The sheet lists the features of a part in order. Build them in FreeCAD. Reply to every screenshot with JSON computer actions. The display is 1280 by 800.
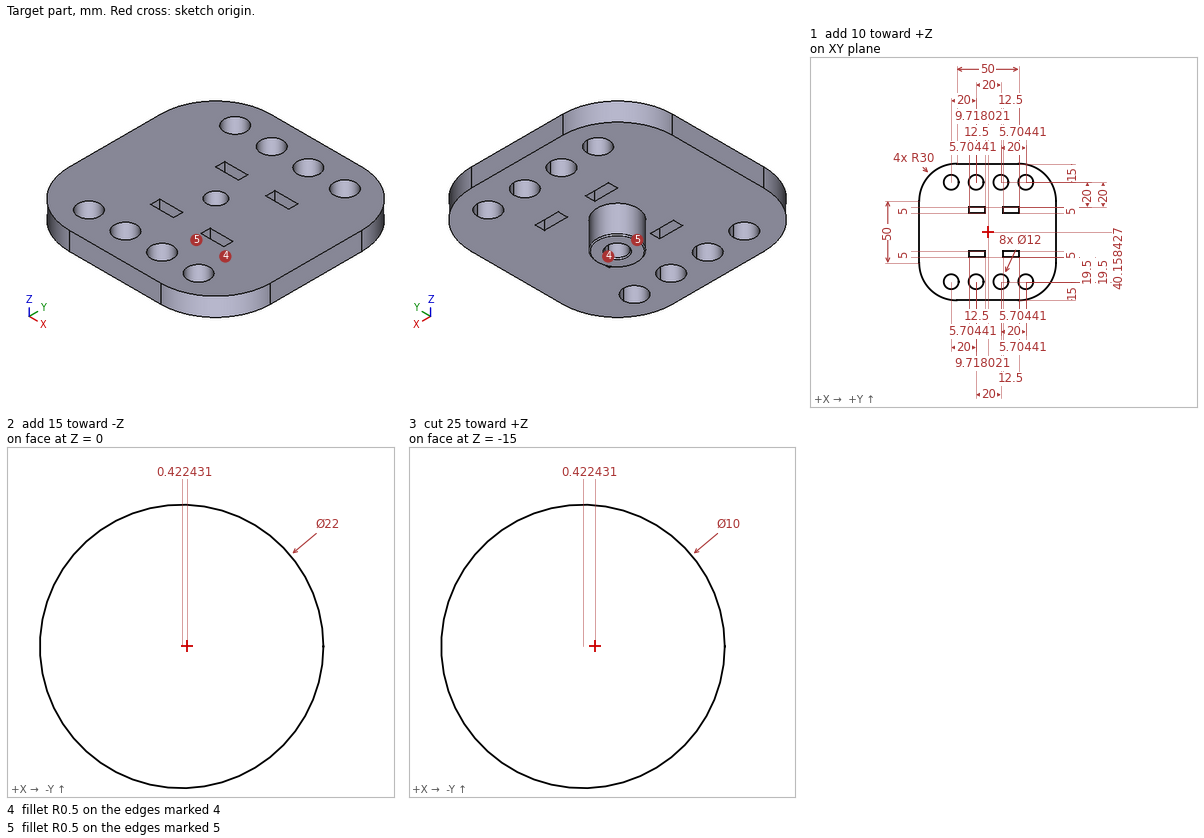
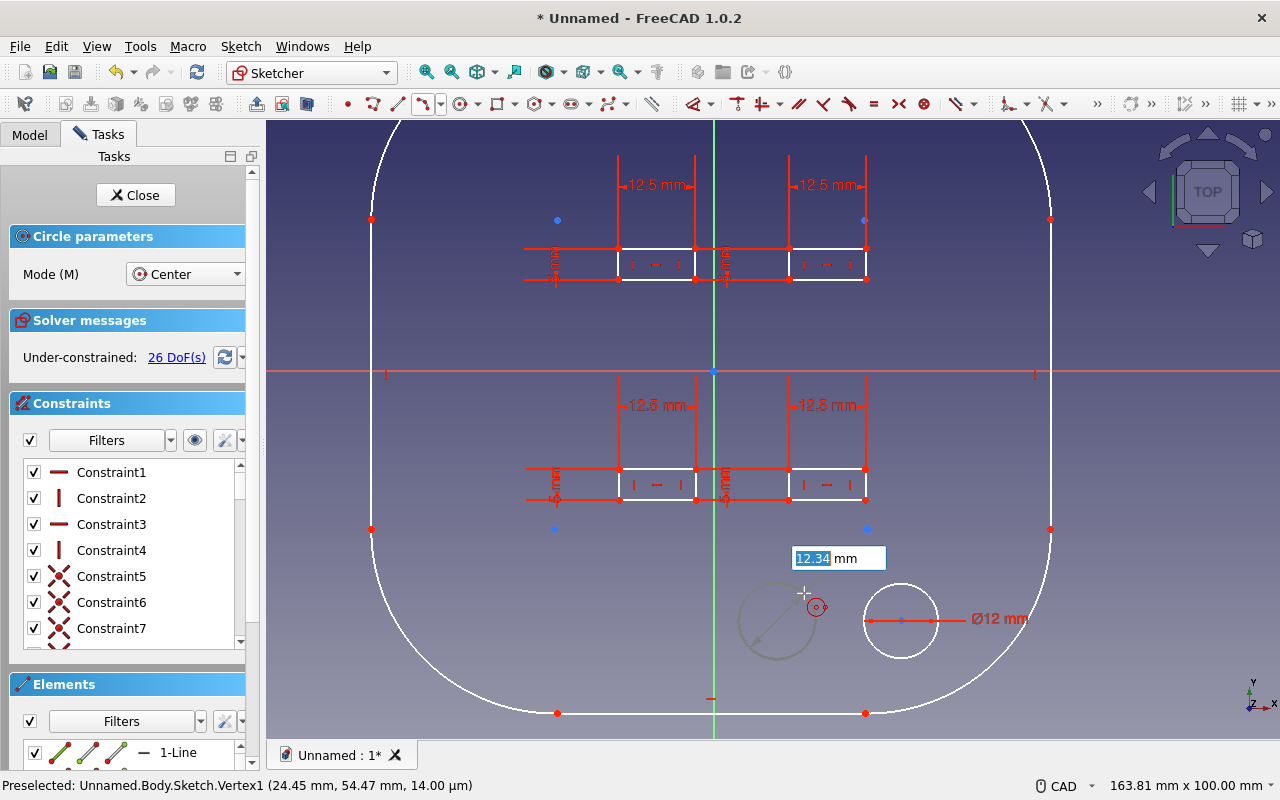
{"action": "type", "text": "12"}
{"action": "key", "text": "Return"}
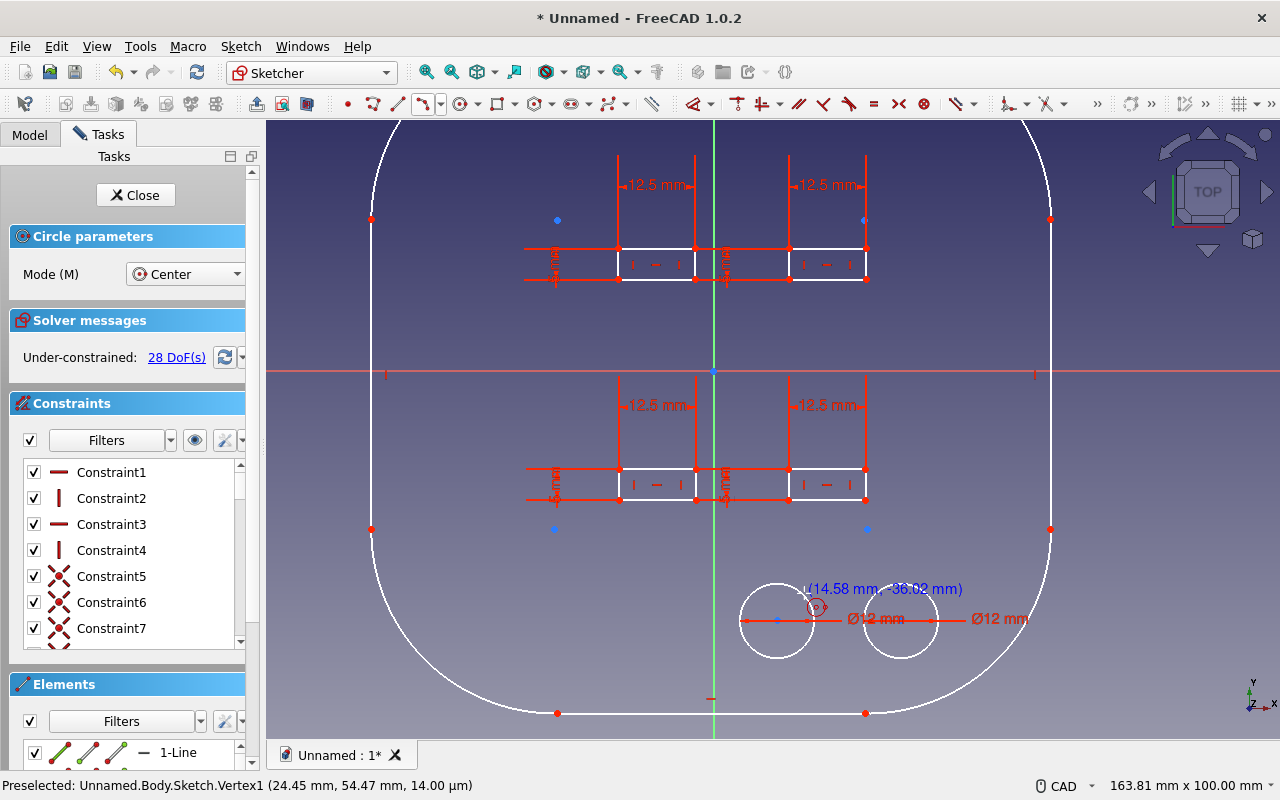
{"action": "left_click", "coordinate": [654, 620]}
{"action": "mouse_move", "coordinate": [680, 593]}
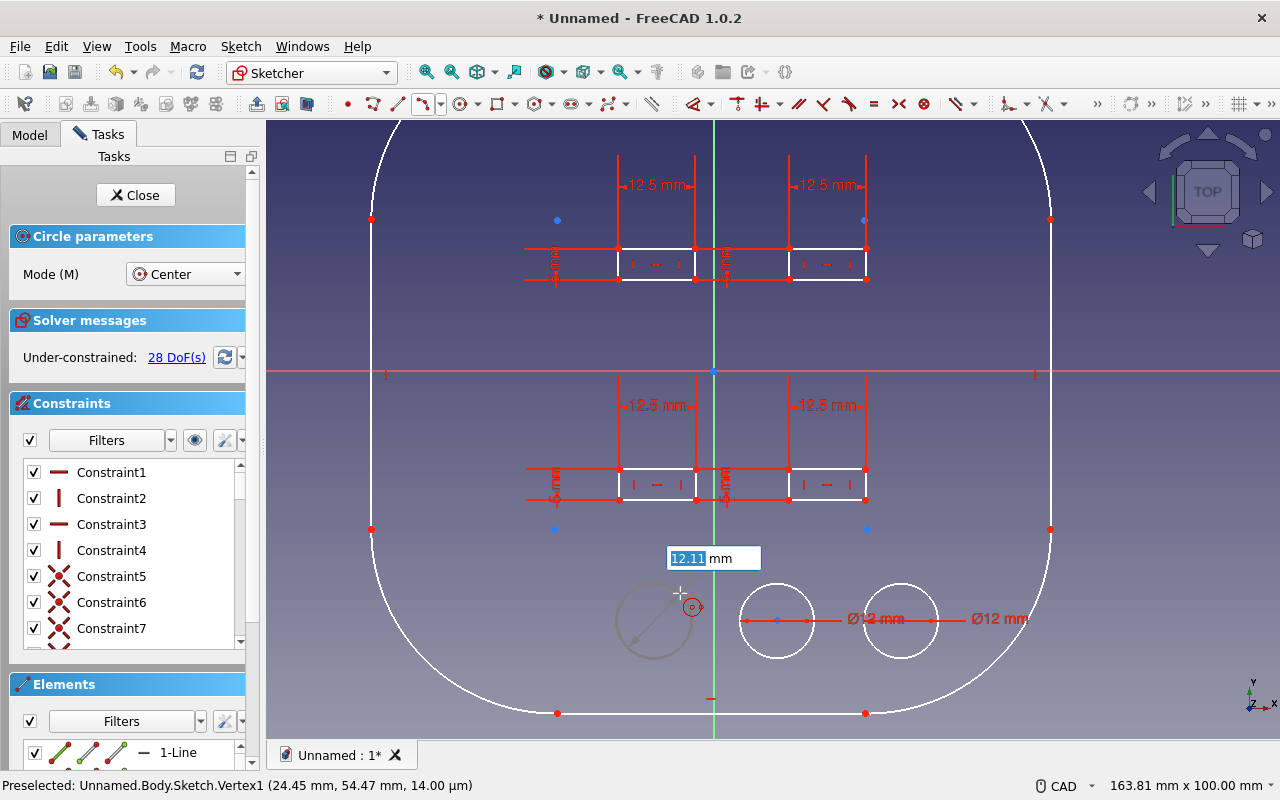
{"action": "type", "text": "12"}
{"action": "key", "text": "Return"}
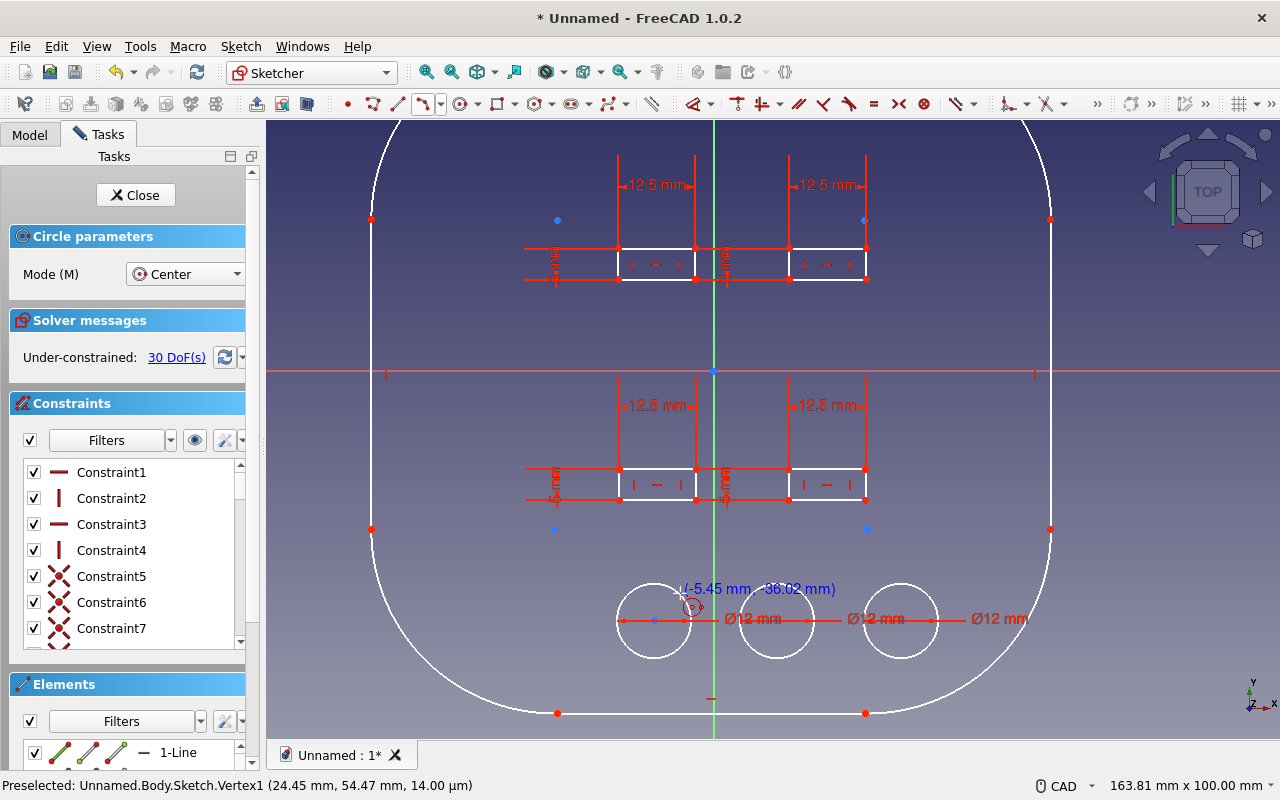
{"action": "left_click", "coordinate": [530, 620]}
{"action": "mouse_move", "coordinate": [556, 593]}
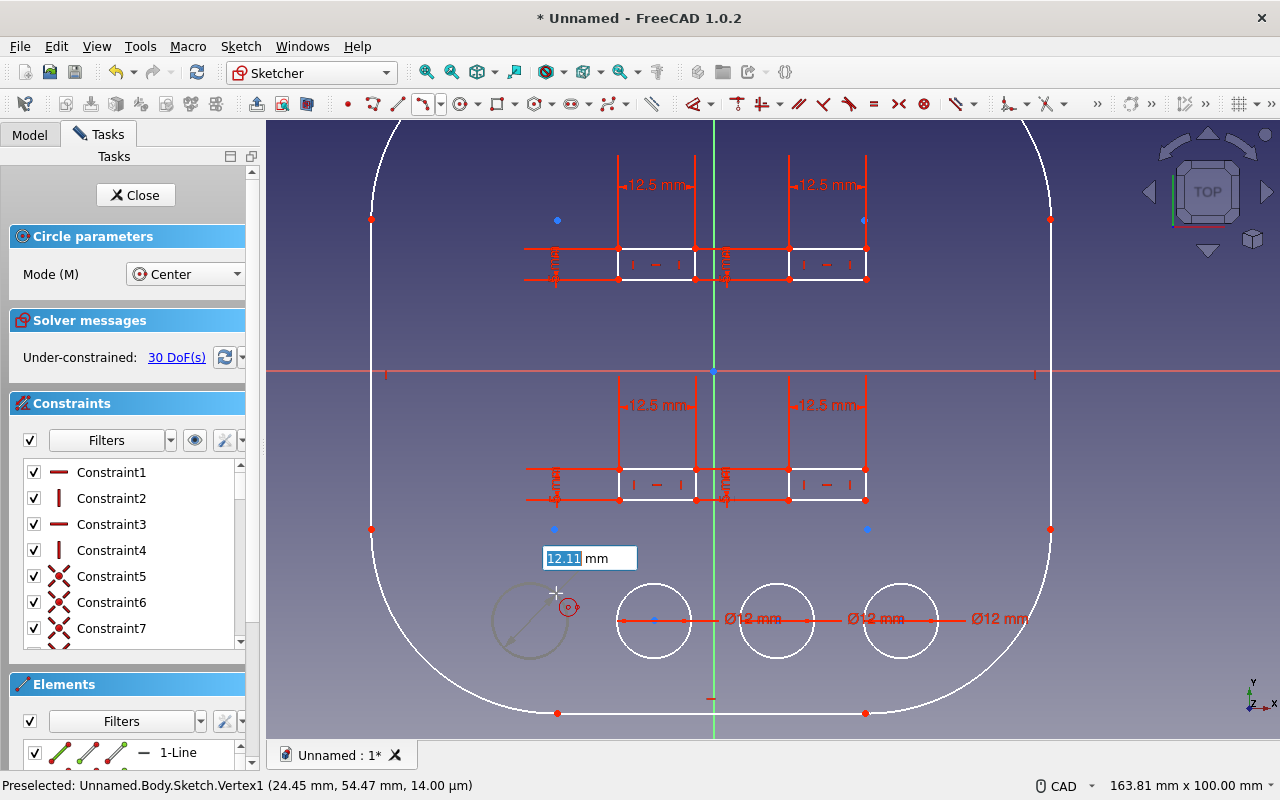
{"action": "type", "text": "12"}
{"action": "key", "text": "Return"}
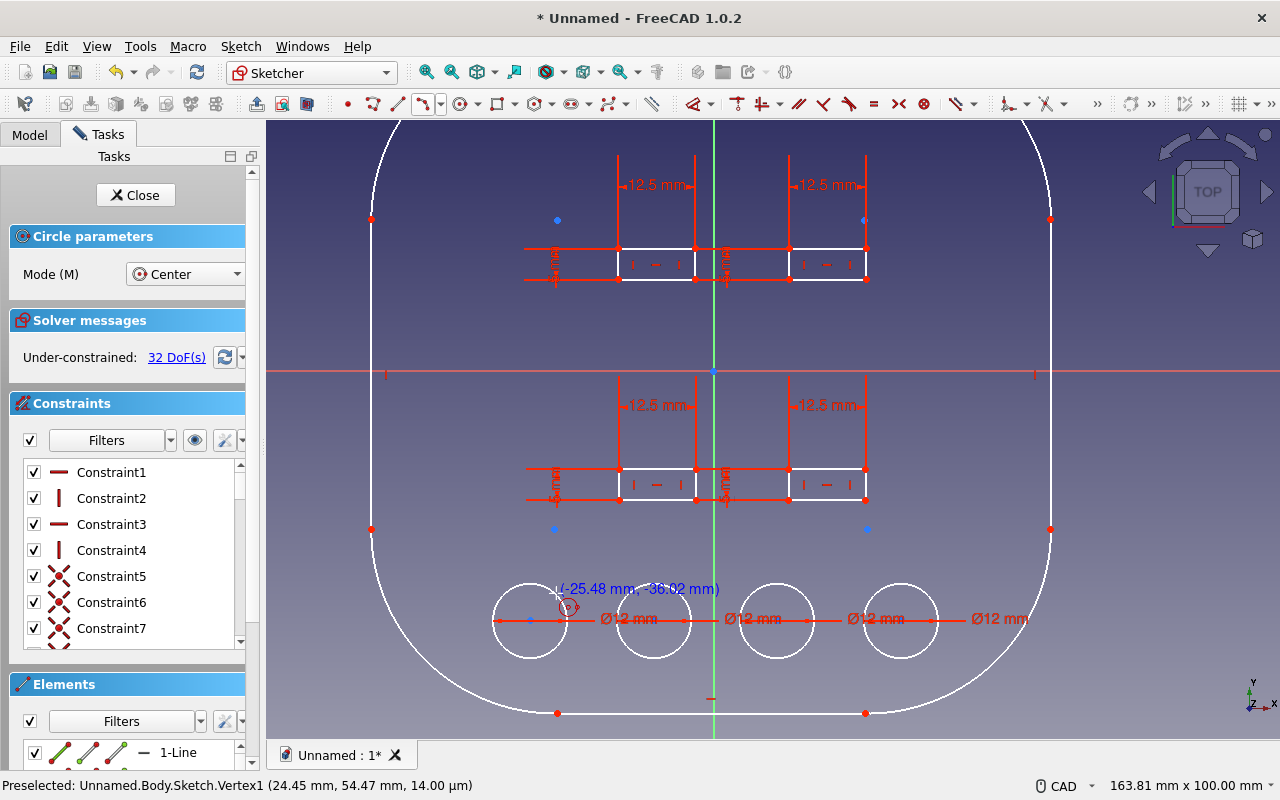
{"action": "scroll", "coordinate": [696, 499], "scroll_direction": "down", "scroll_amount": 3}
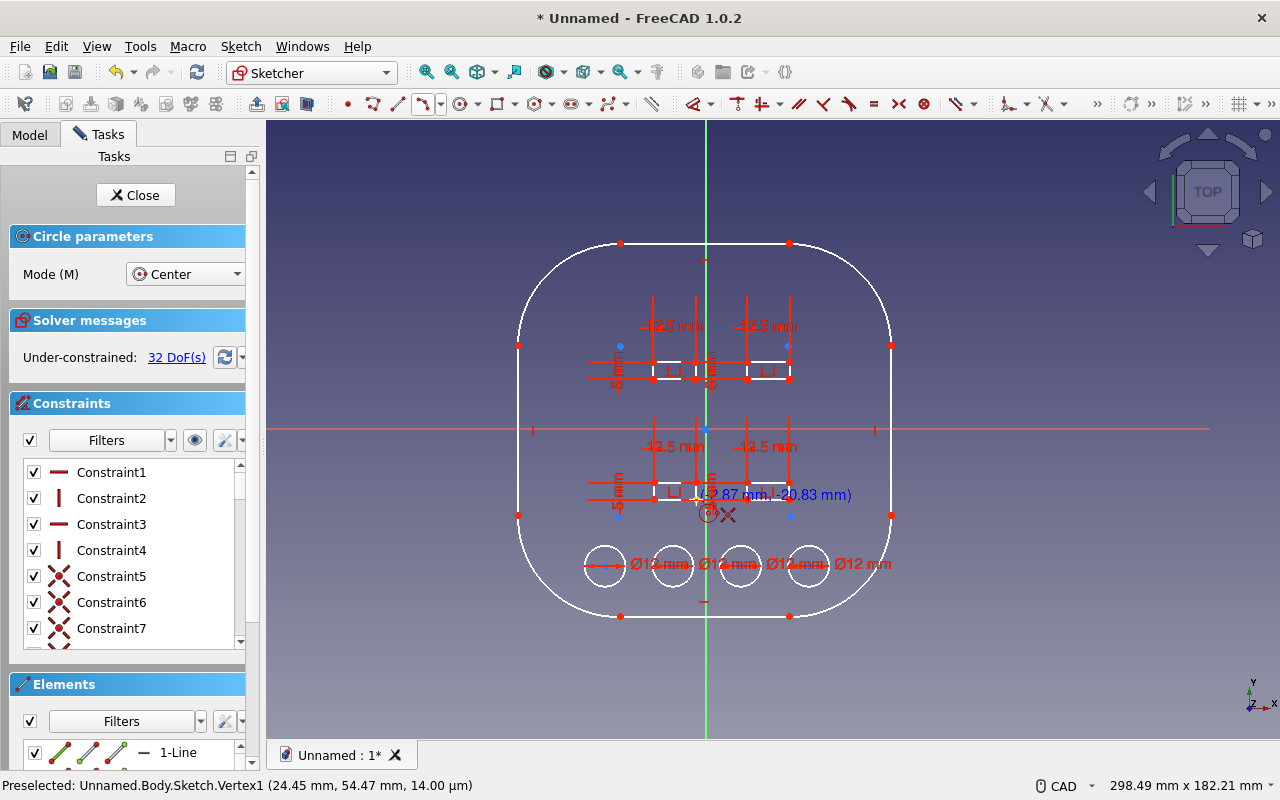
{"action": "left_click", "coordinate": [809, 294]}
{"action": "mouse_move", "coordinate": [823, 279]}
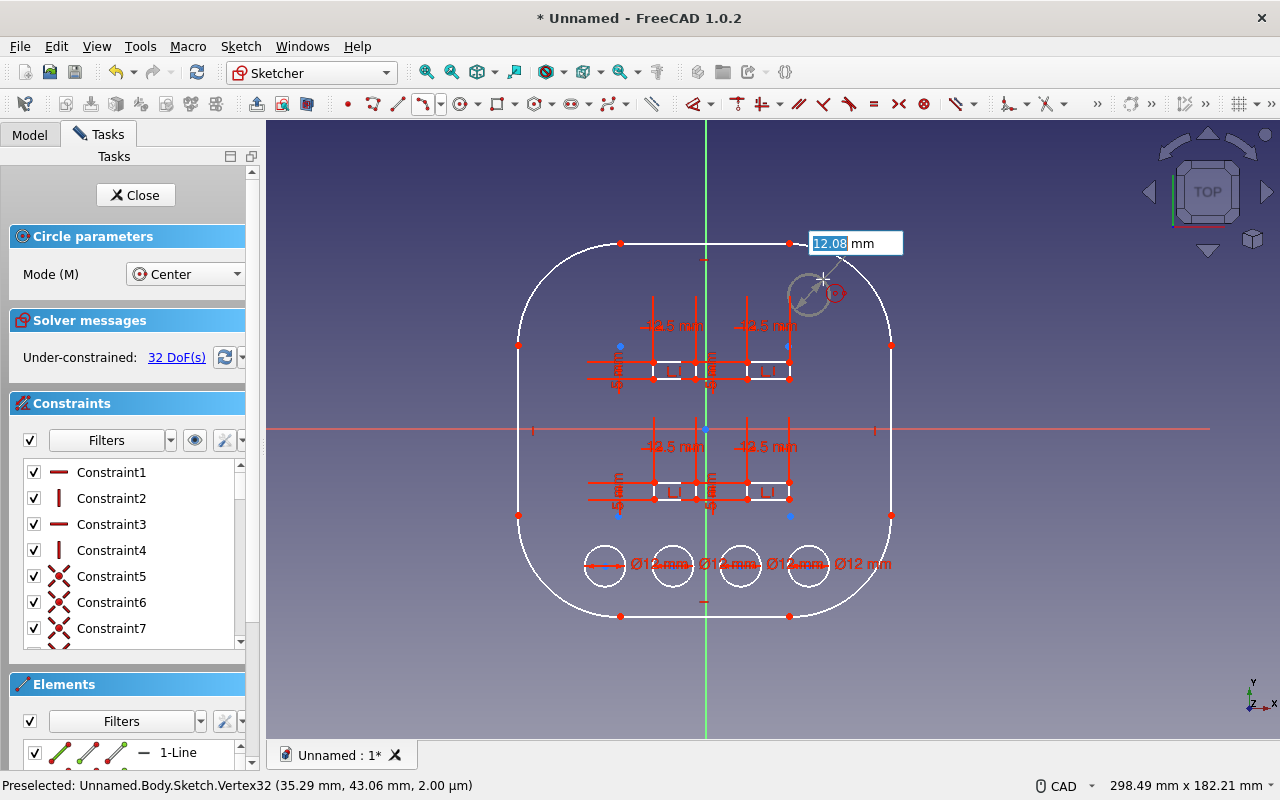
{"action": "type", "text": "12"}
{"action": "key", "text": "Return"}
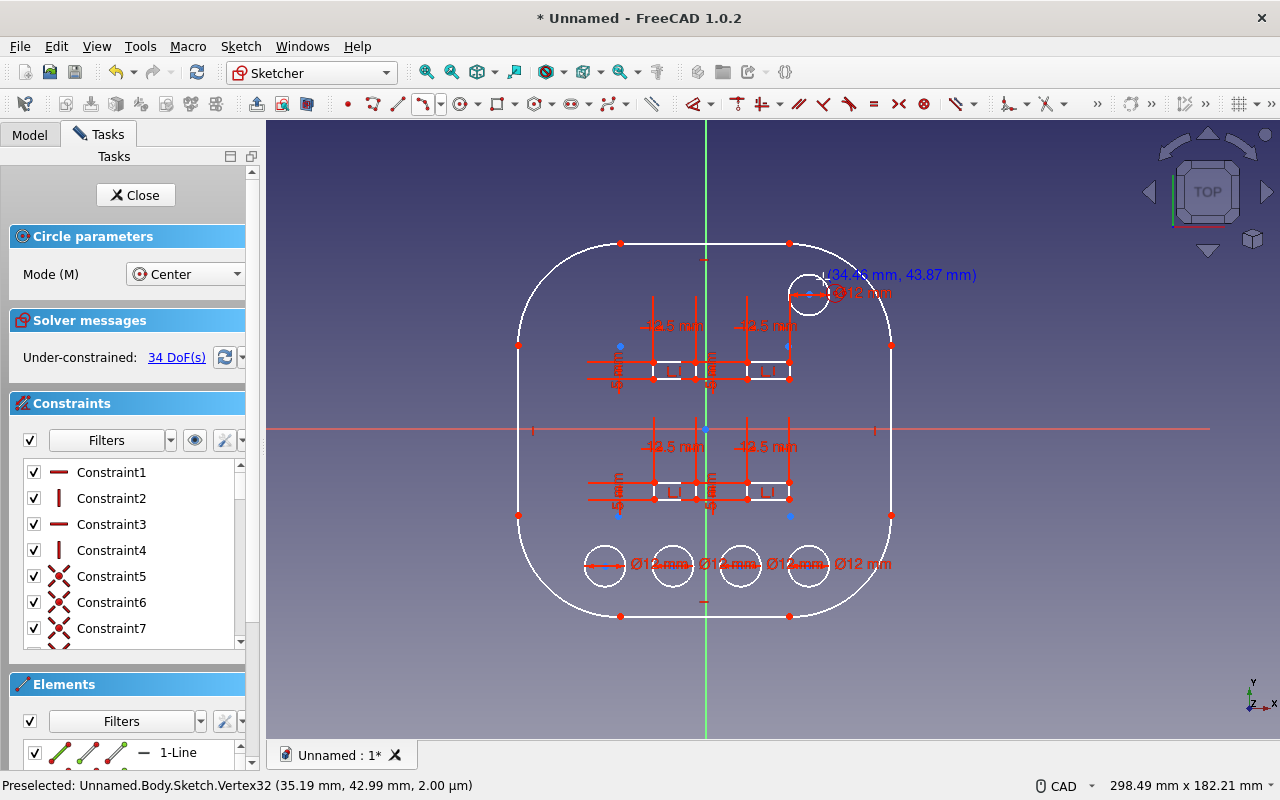
{"action": "left_click", "coordinate": [741, 294]}
{"action": "mouse_move", "coordinate": [755, 279]}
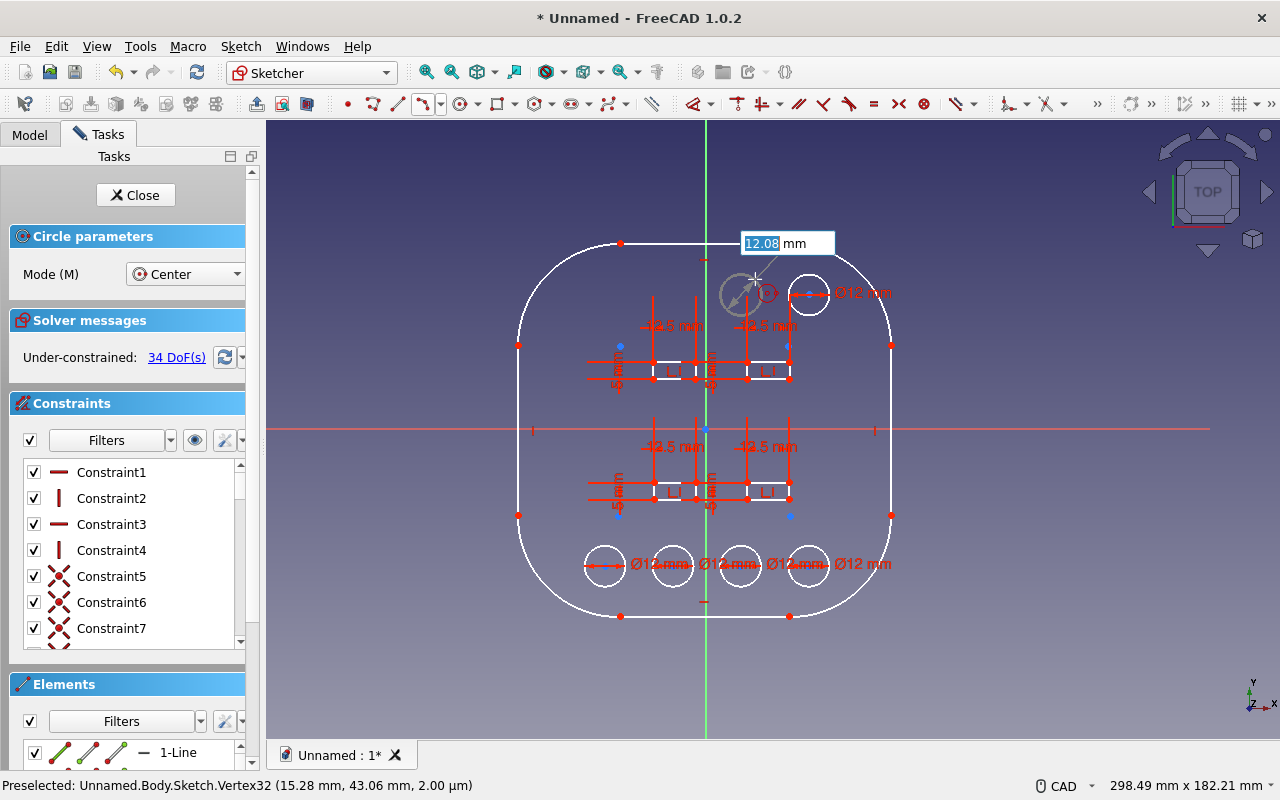
{"action": "type", "text": "12"}
{"action": "key", "text": "Return"}